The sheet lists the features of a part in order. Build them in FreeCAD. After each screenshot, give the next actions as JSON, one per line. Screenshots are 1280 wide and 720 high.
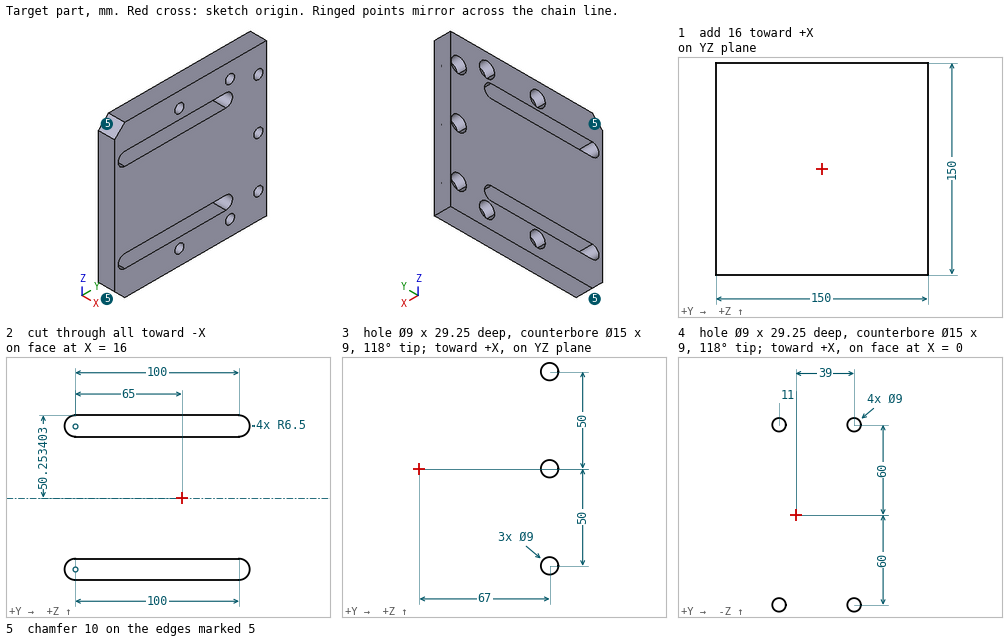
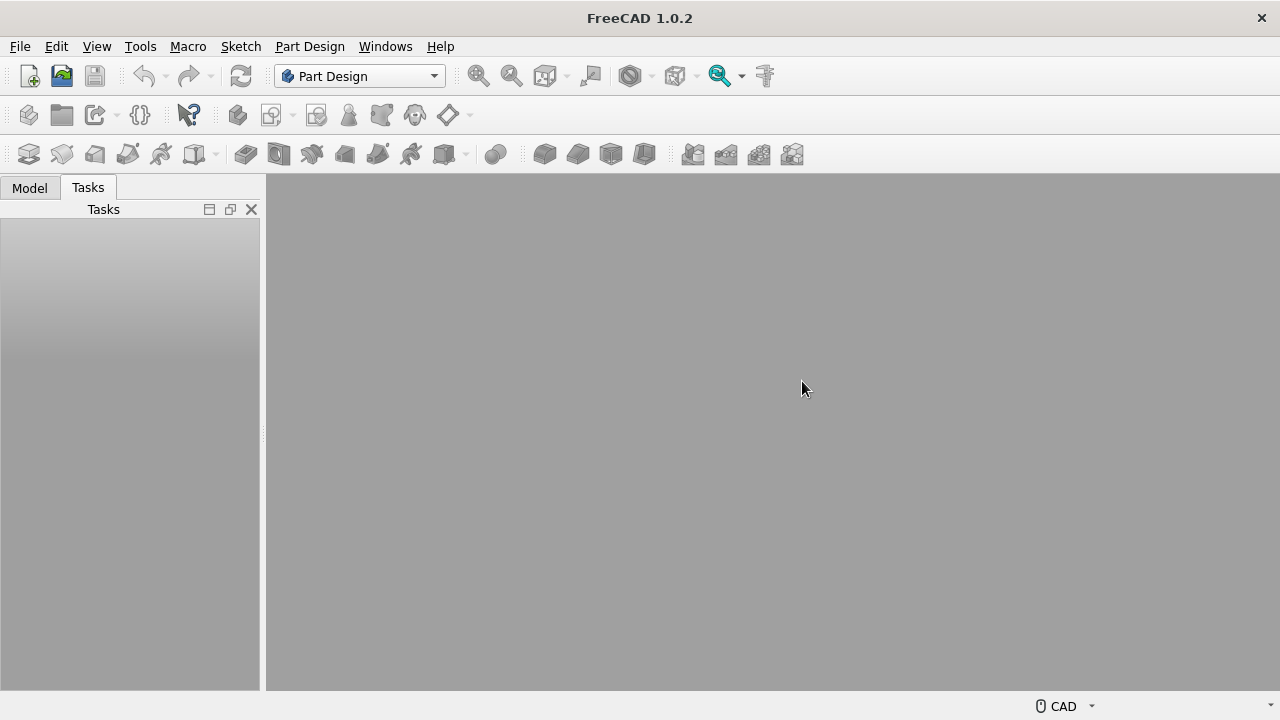
{"action": "left_click", "coordinate": [29, 76]}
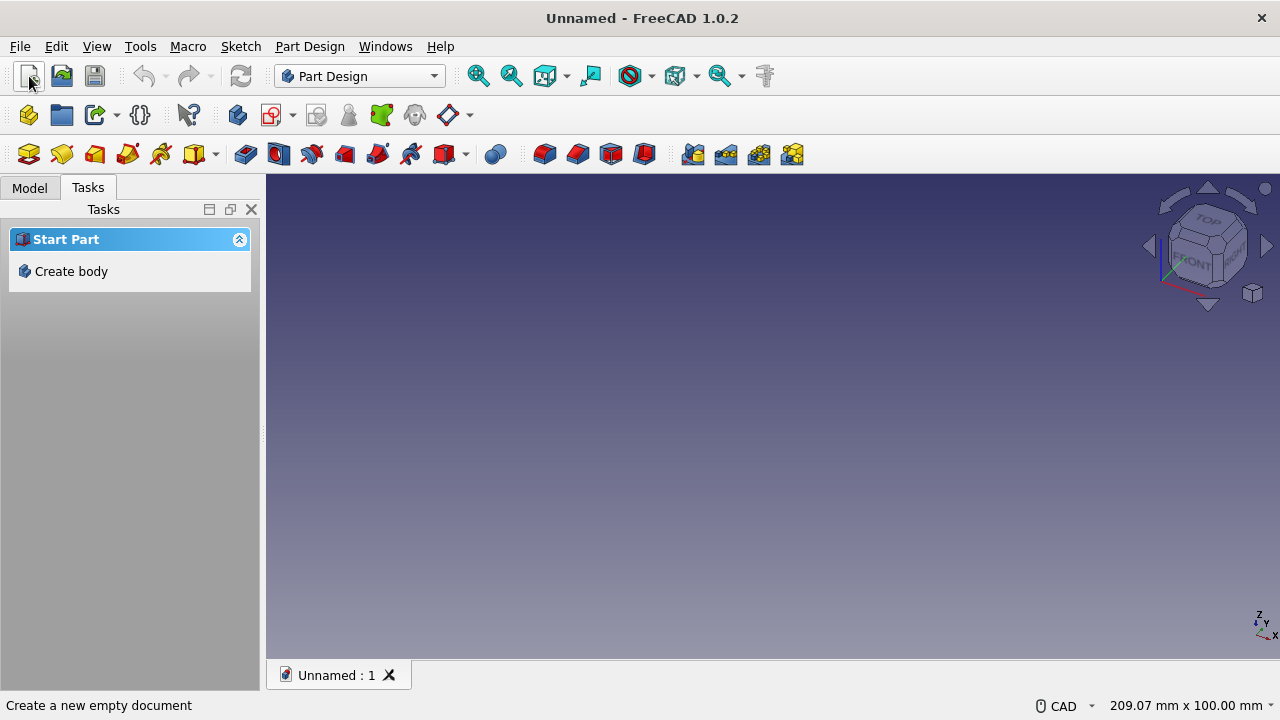
{"action": "left_click", "coordinate": [270, 116]}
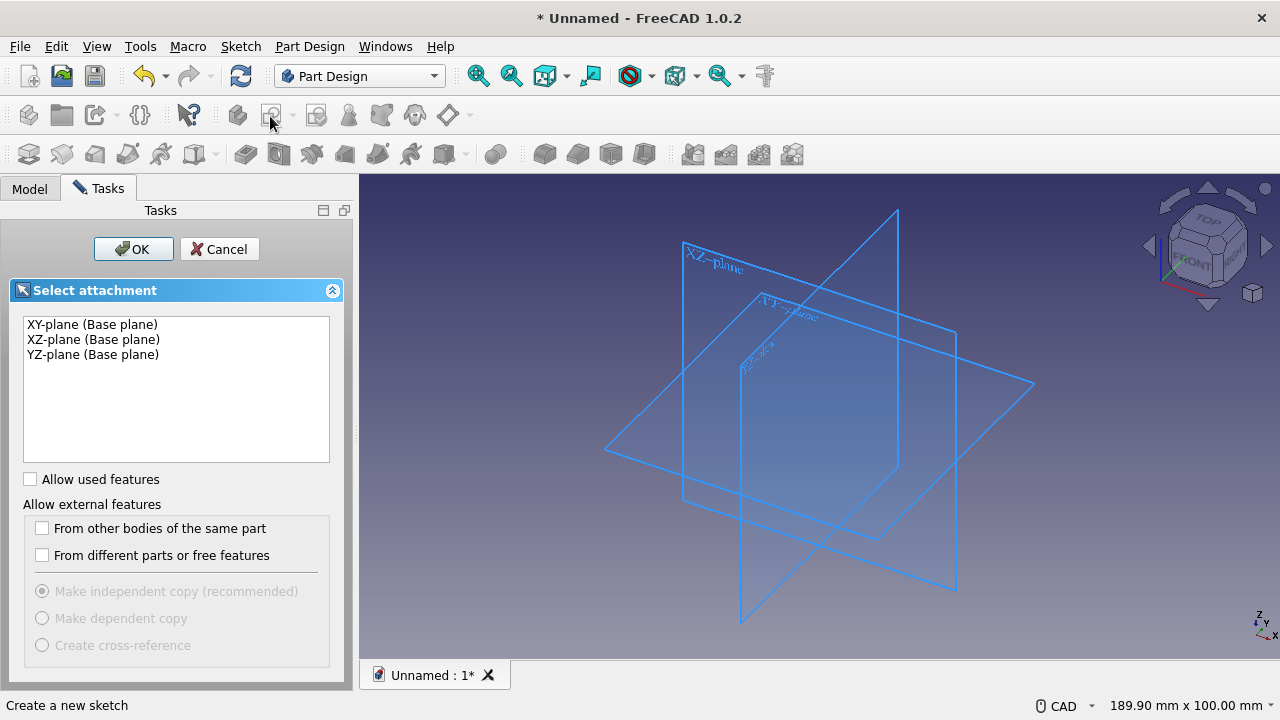
{"action": "left_click", "coordinate": [84, 354]}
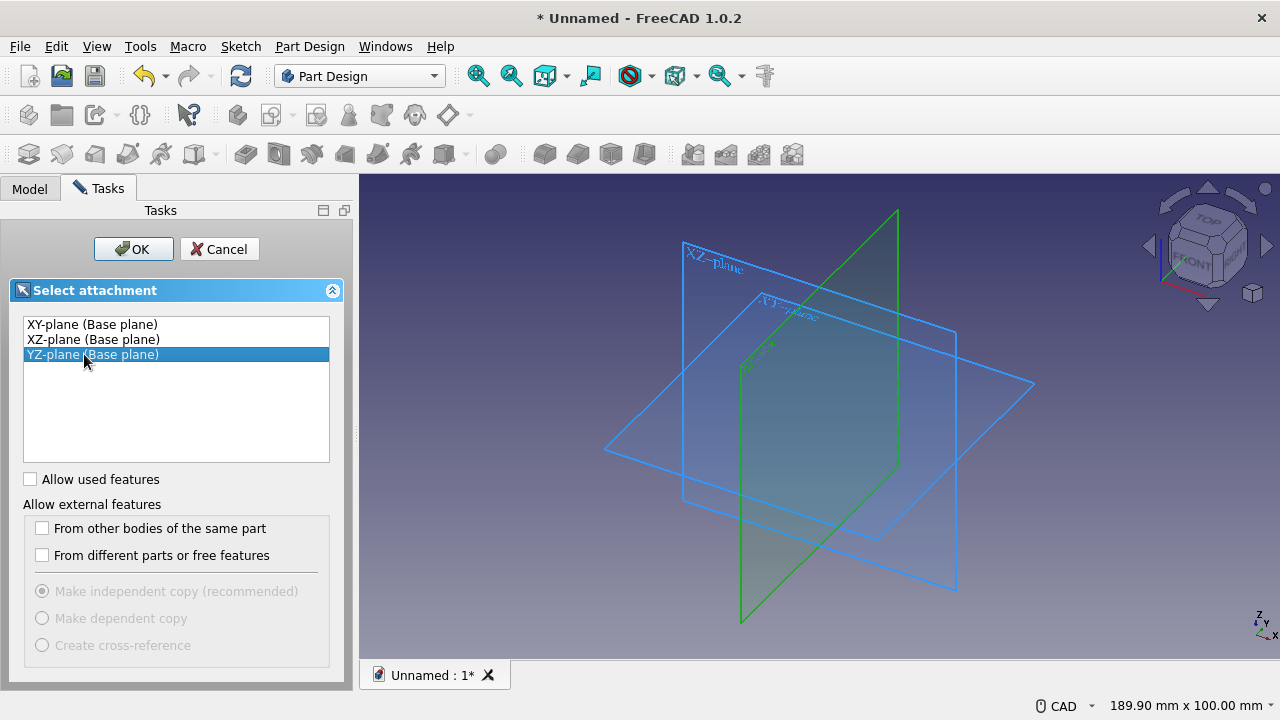
{"action": "left_click", "coordinate": [134, 249]}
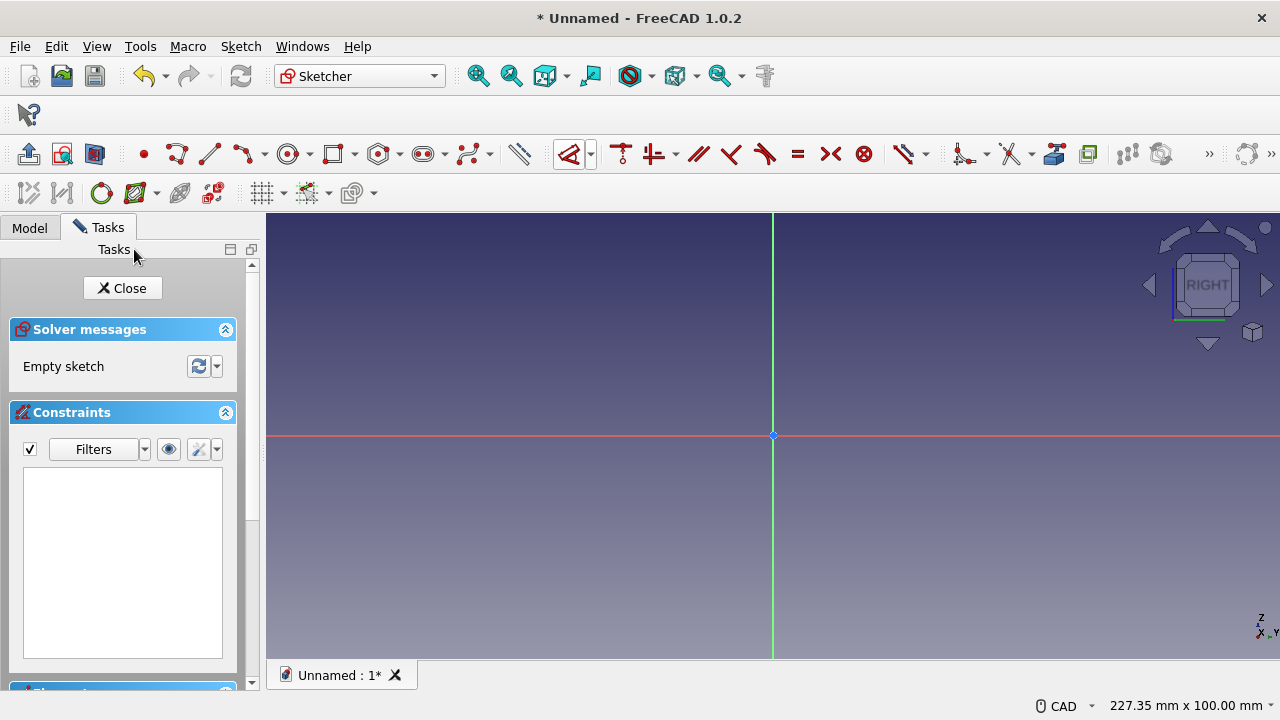
{"action": "scroll", "coordinate": [649, 436], "scroll_direction": "down", "scroll_amount": 4}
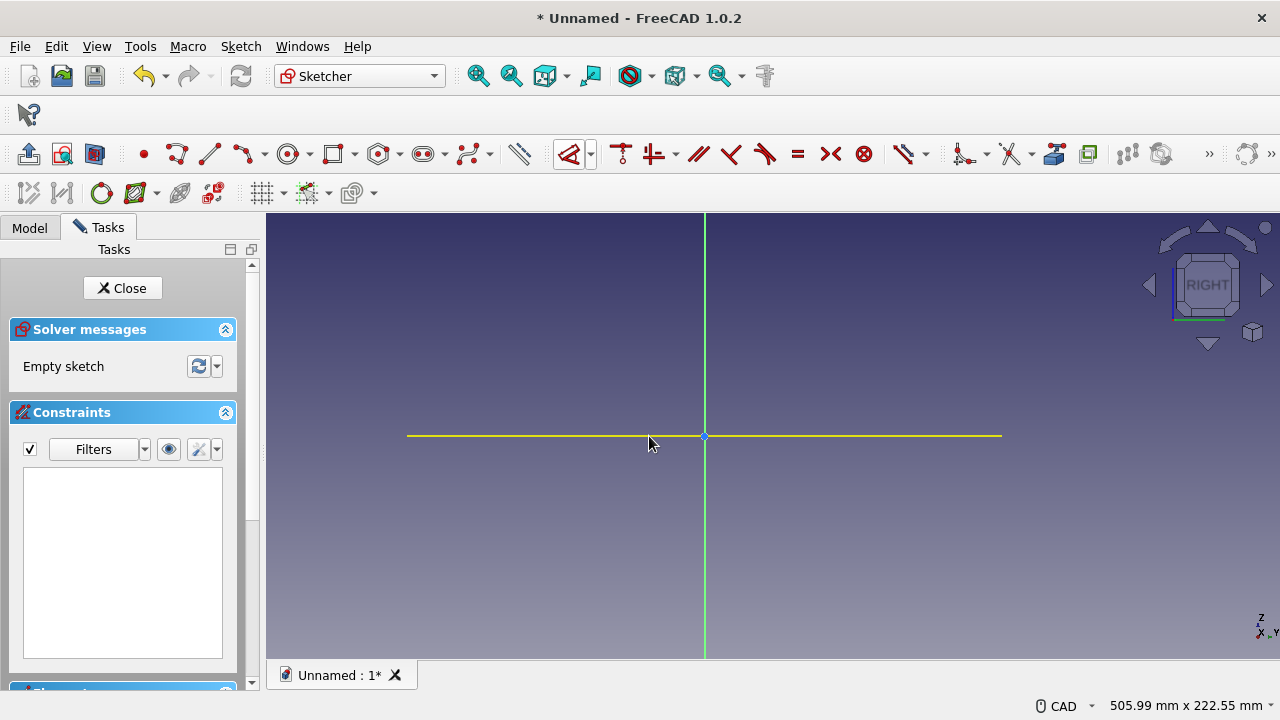
{"action": "left_click", "coordinate": [354, 154]}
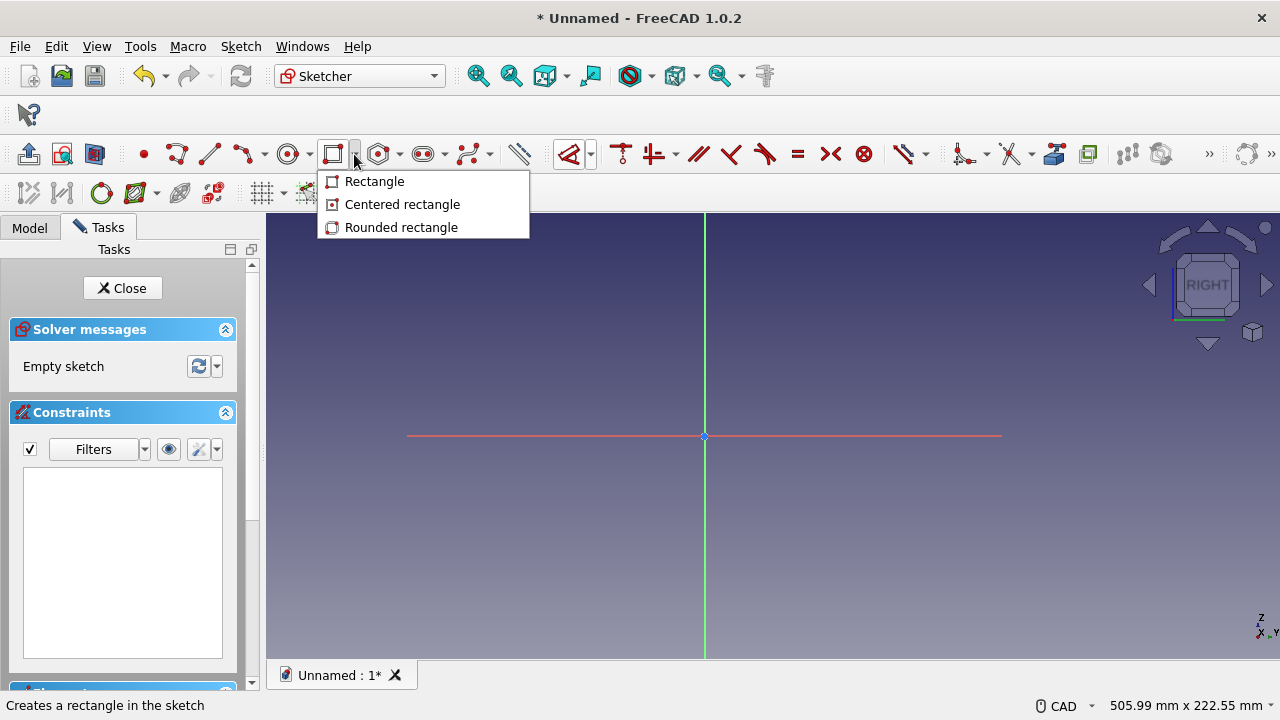
{"action": "left_click", "coordinate": [424, 204]}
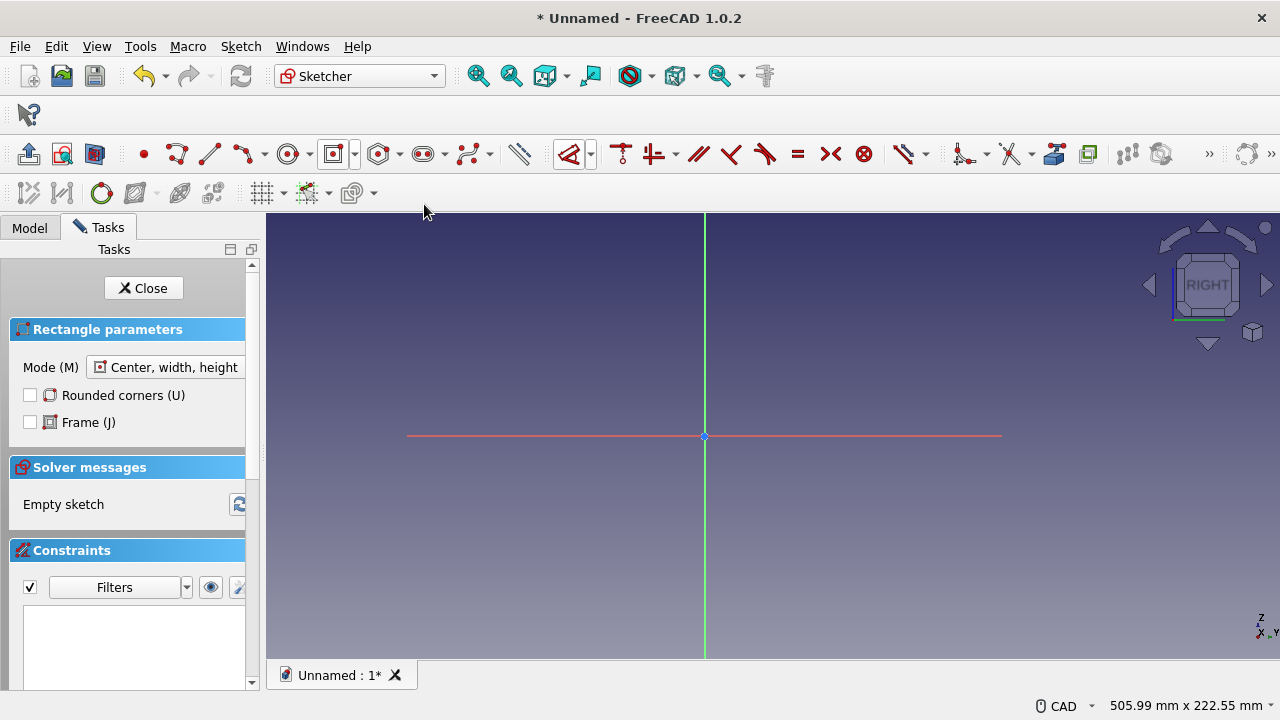
{"action": "left_click", "coordinate": [705, 436]}
{"action": "mouse_move", "coordinate": [855, 286]}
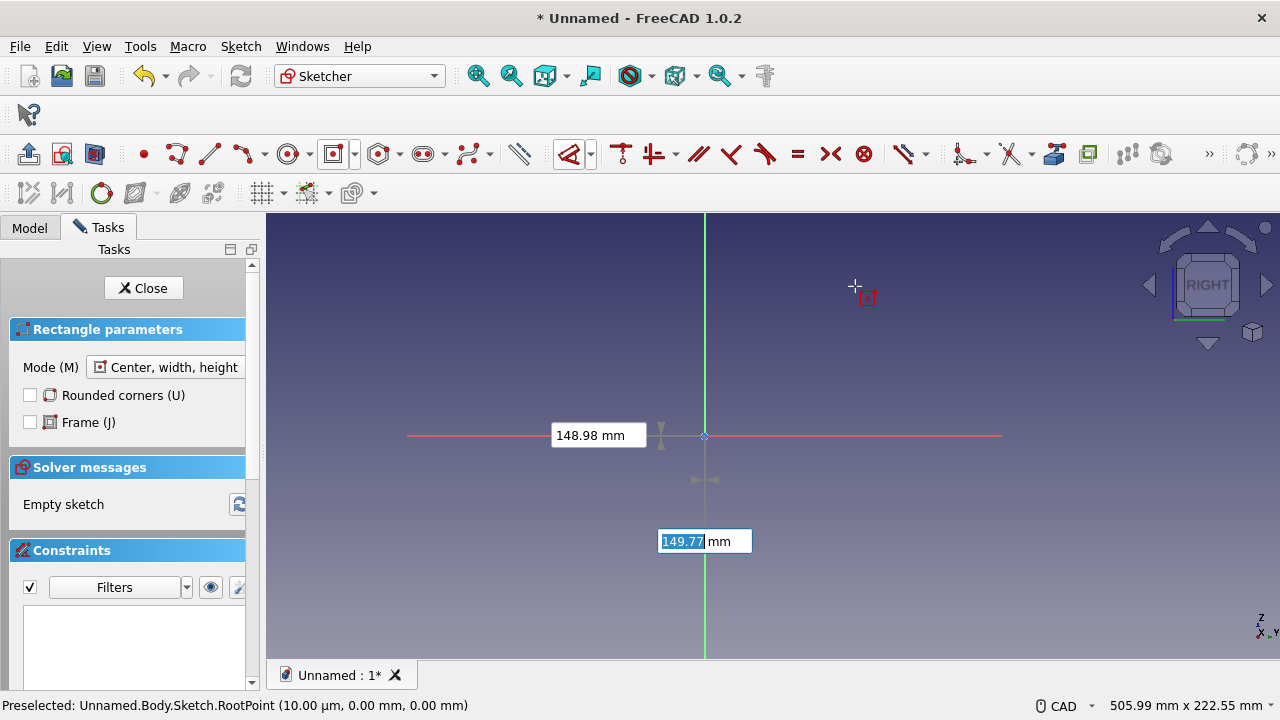
{"action": "type", "text": "150"}
{"action": "key", "text": "Tab"}
{"action": "type", "text": "150"}
{"action": "key", "text": "Return"}
{"action": "key", "text": "Escape"}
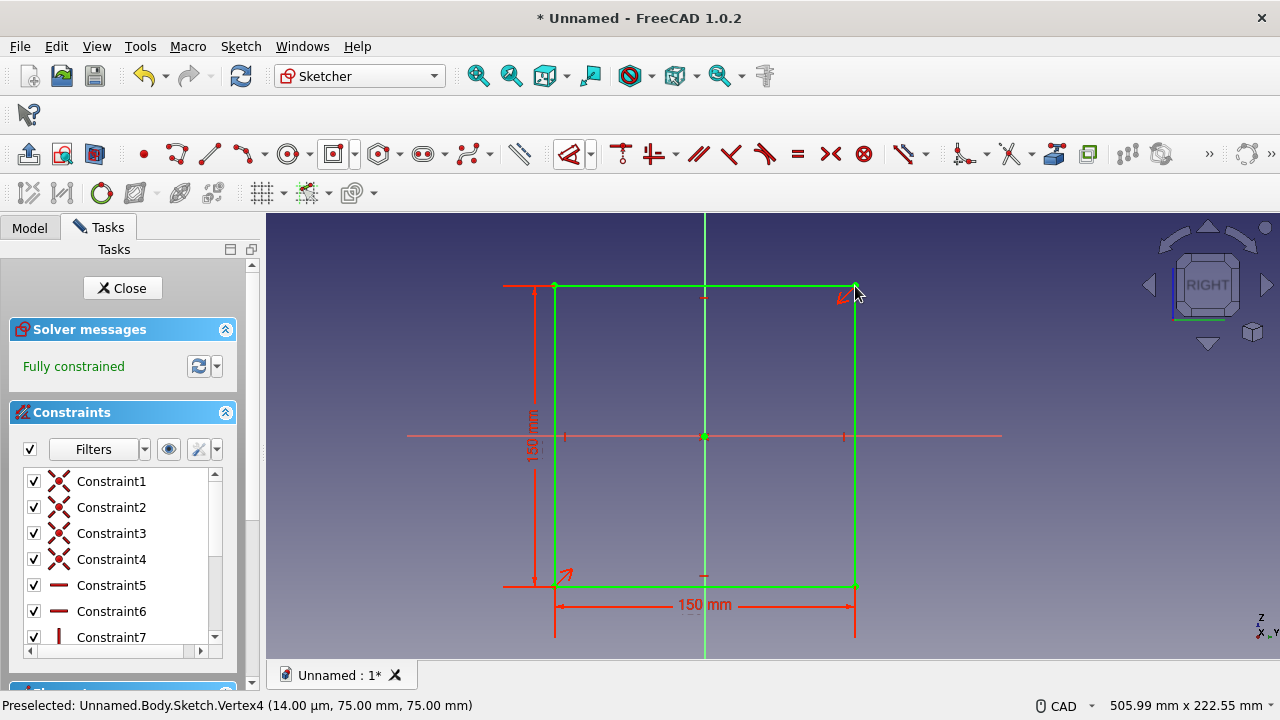
{"action": "left_click", "coordinate": [123, 288]}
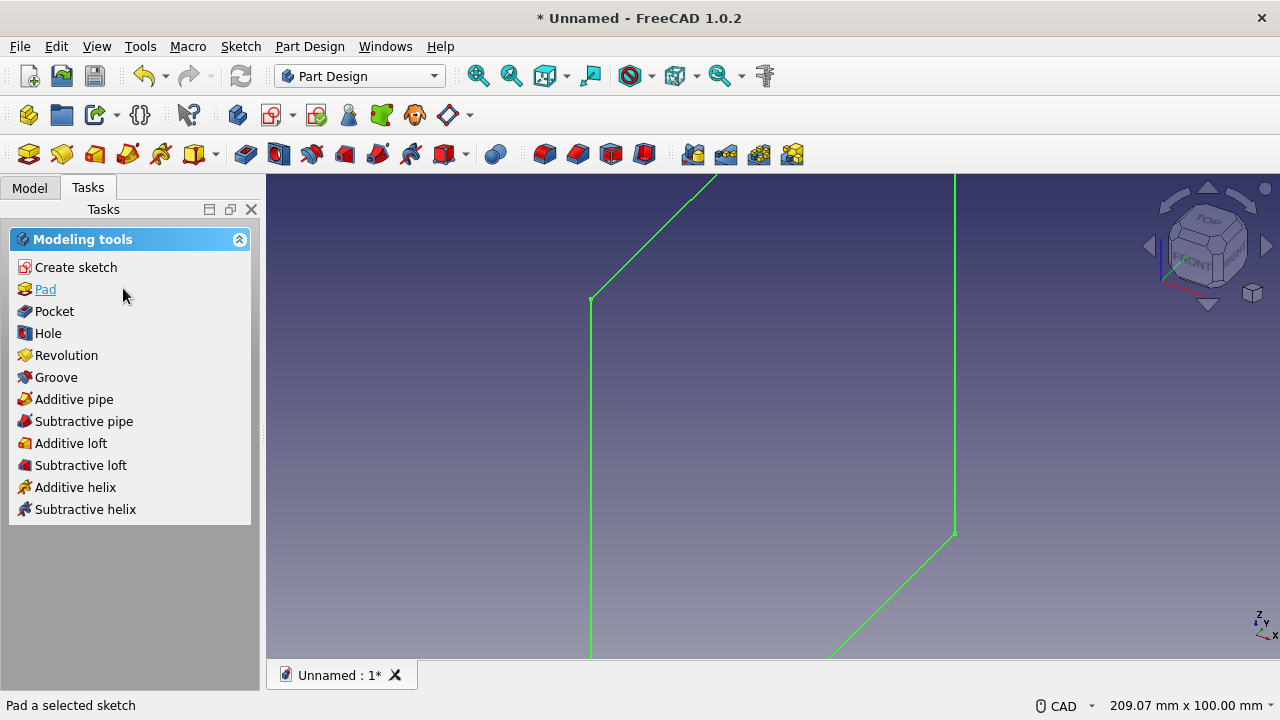
{"action": "left_click", "coordinate": [29, 154]}